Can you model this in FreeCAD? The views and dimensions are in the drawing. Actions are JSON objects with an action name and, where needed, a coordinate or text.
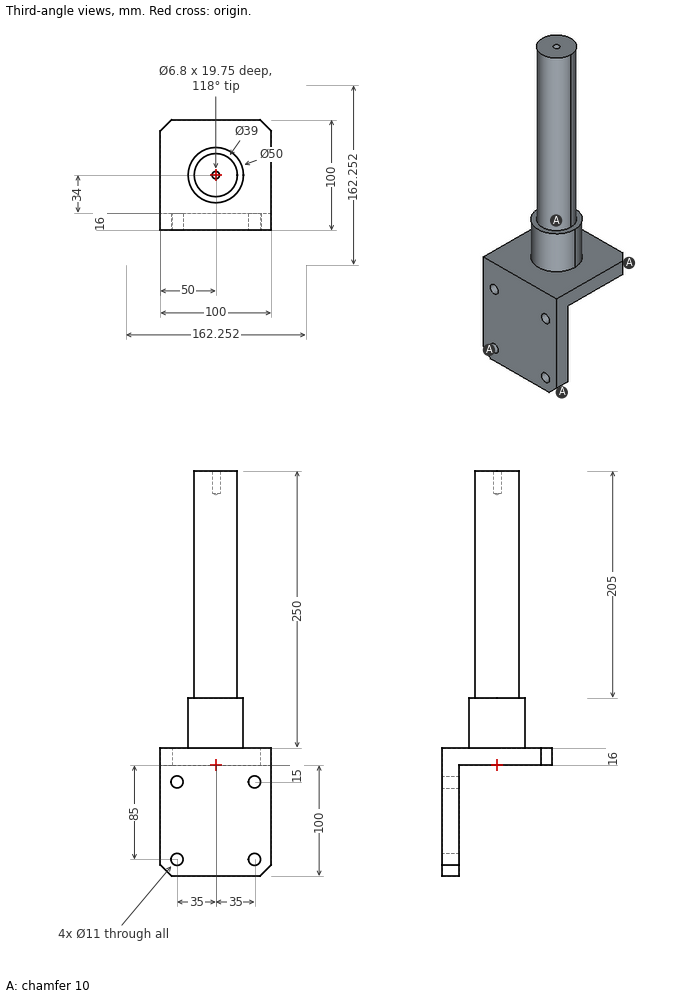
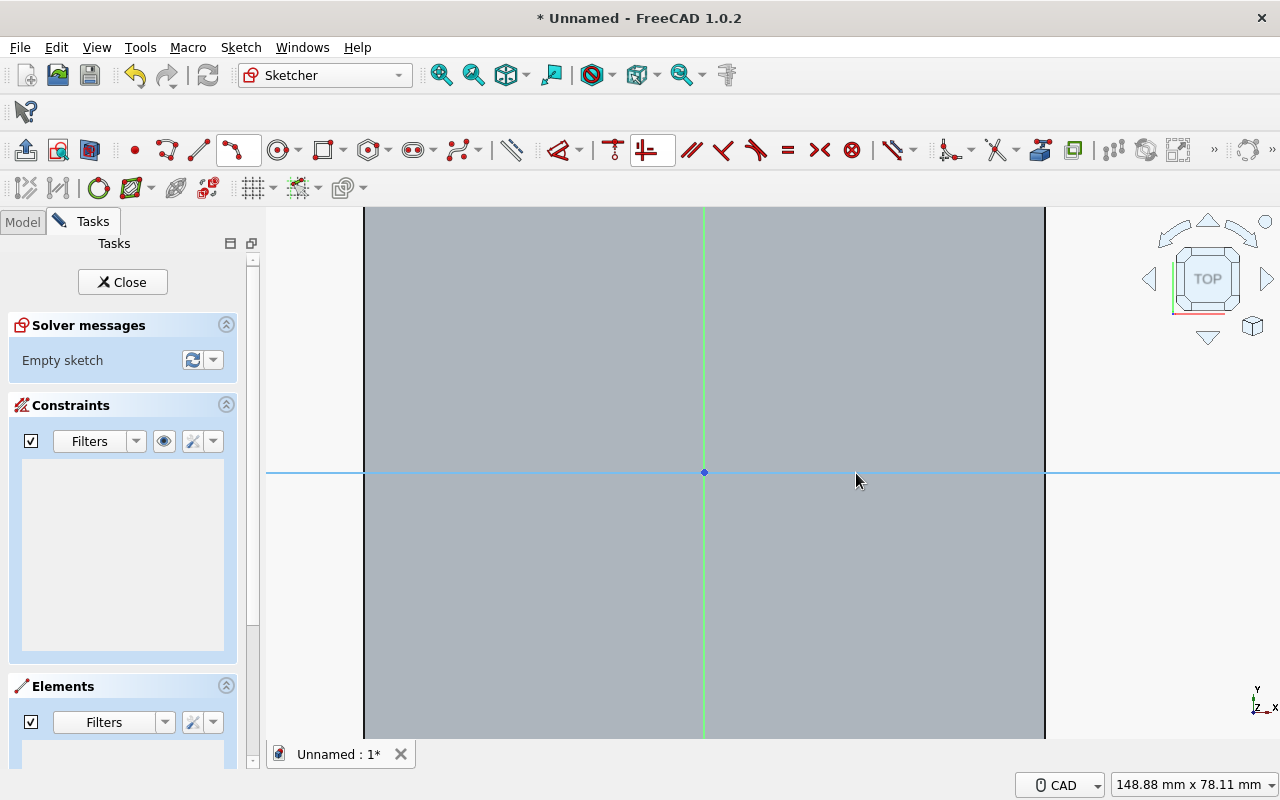
{"action": "left_click", "coordinate": [278, 150]}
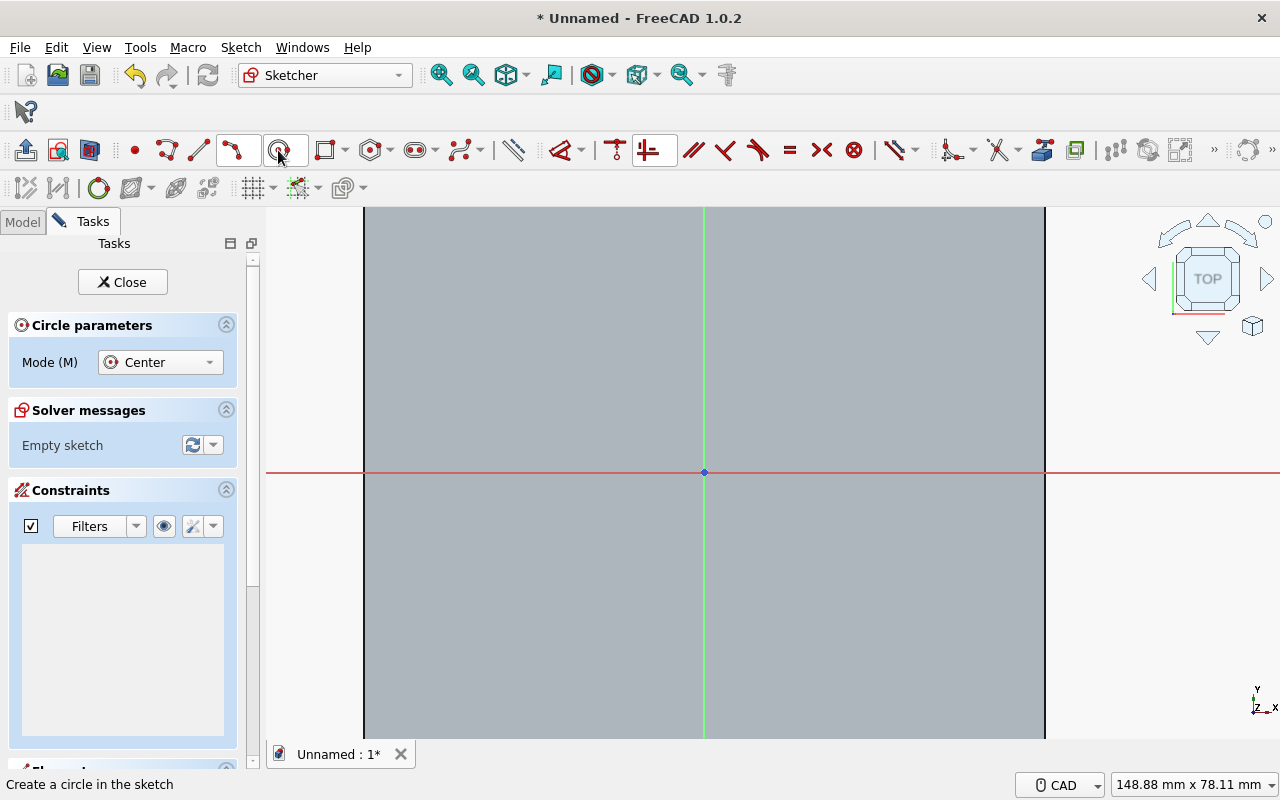
{"action": "left_click", "coordinate": [704, 473]}
{"action": "left_click", "coordinate": [825, 352]}
{"action": "key", "text": "Escape"}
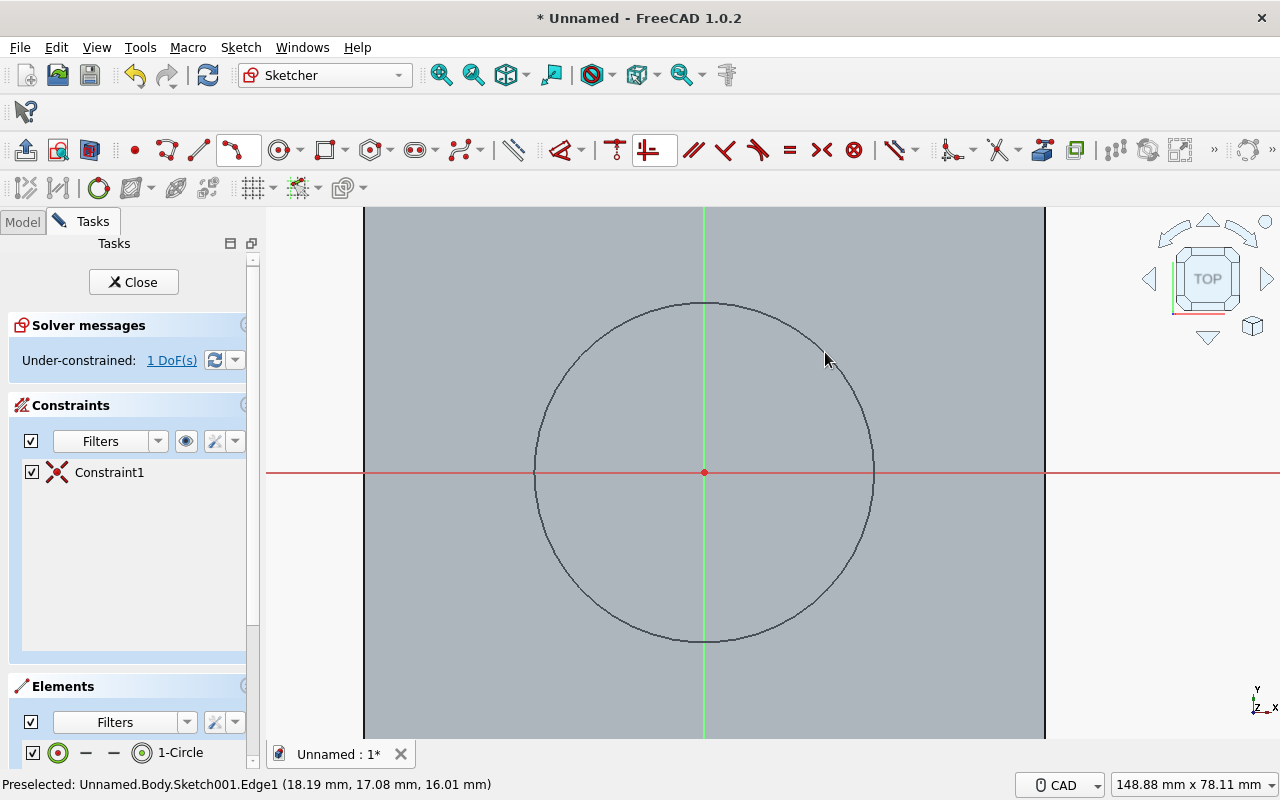
{"action": "left_click", "coordinate": [560, 150]}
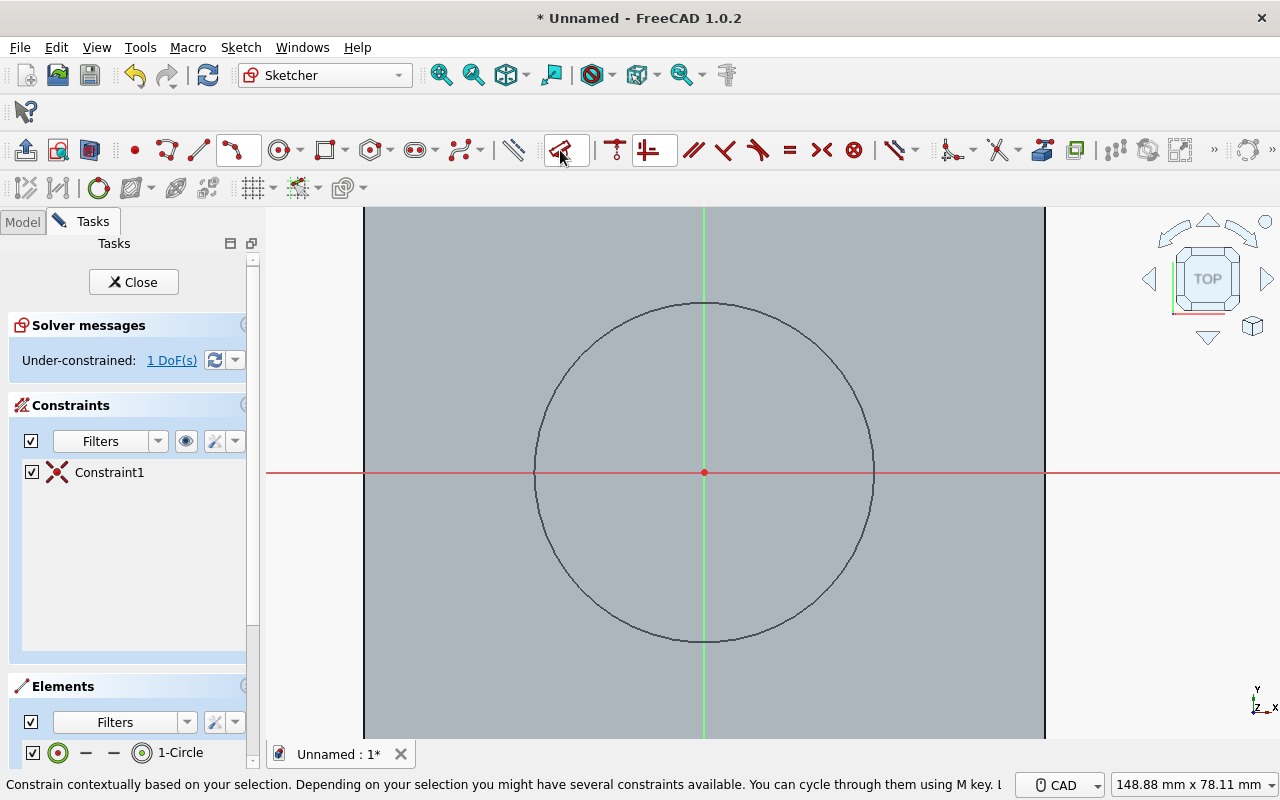
{"action": "left_click", "coordinate": [824, 352]}
{"action": "left_click", "coordinate": [847, 329]}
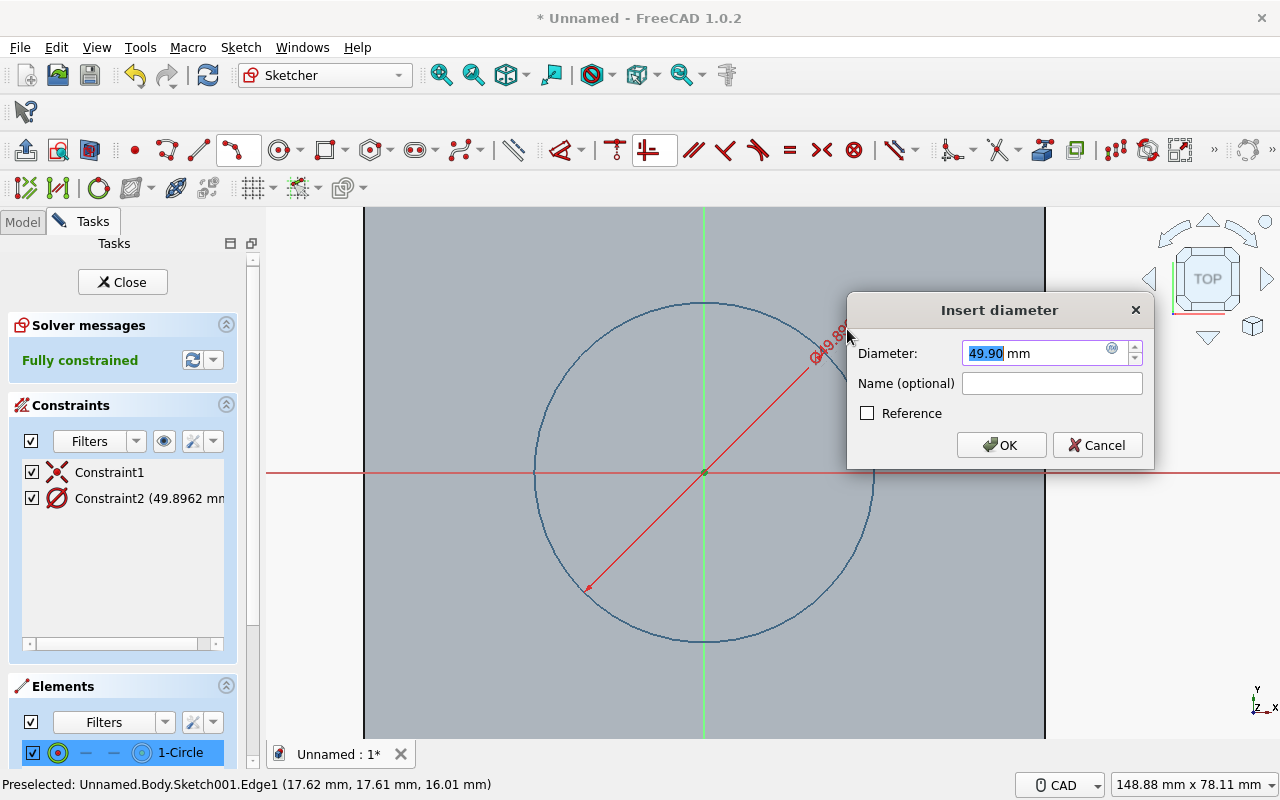
{"action": "type", "text": "50"}
{"action": "key", "text": "Return"}
{"action": "key", "text": "Escape"}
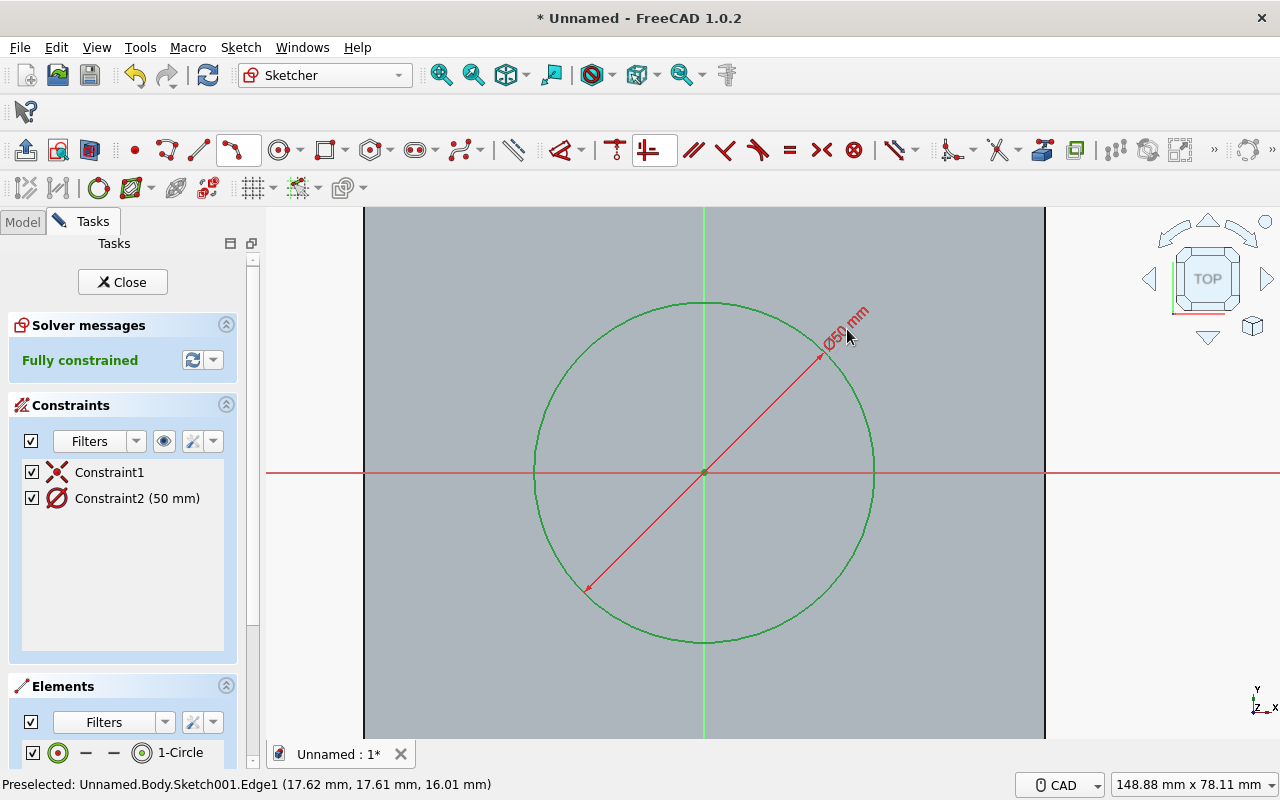
{"action": "left_click", "coordinate": [123, 282]}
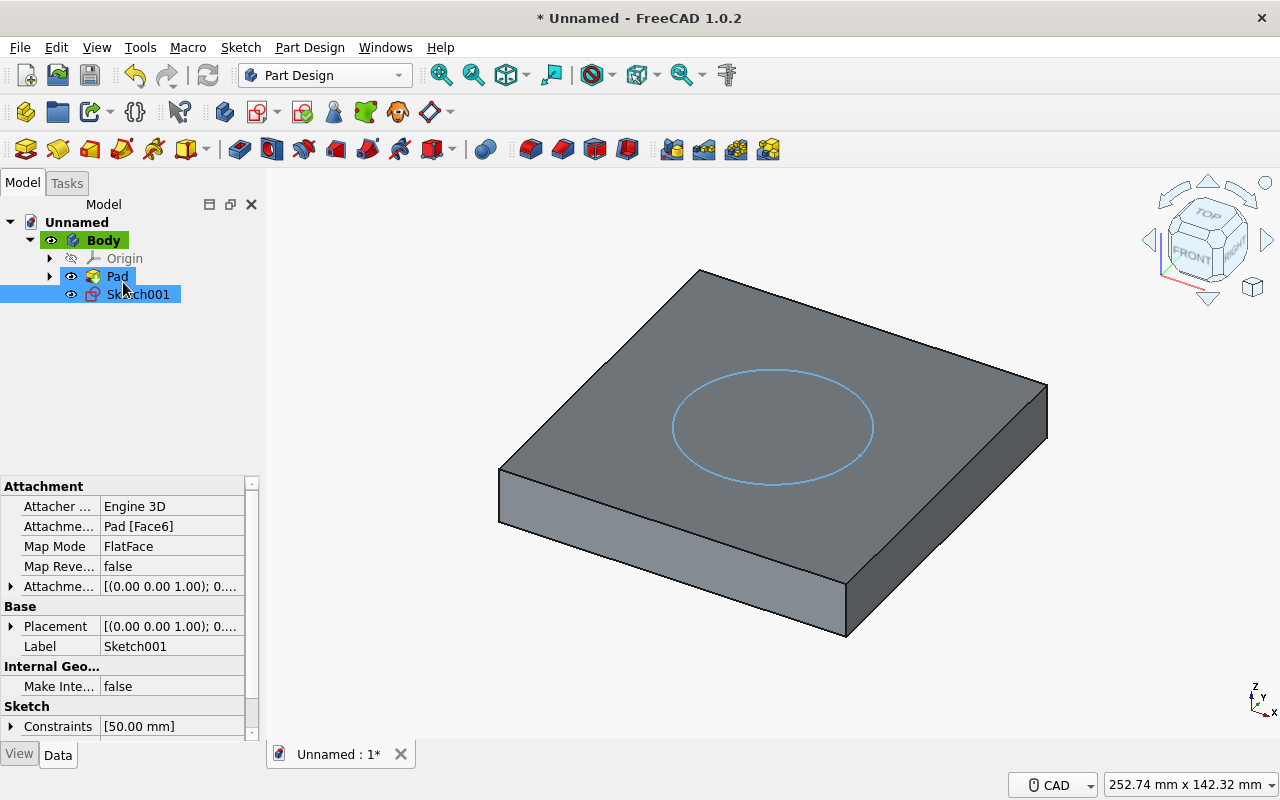
{"action": "left_click", "coordinate": [26, 150]}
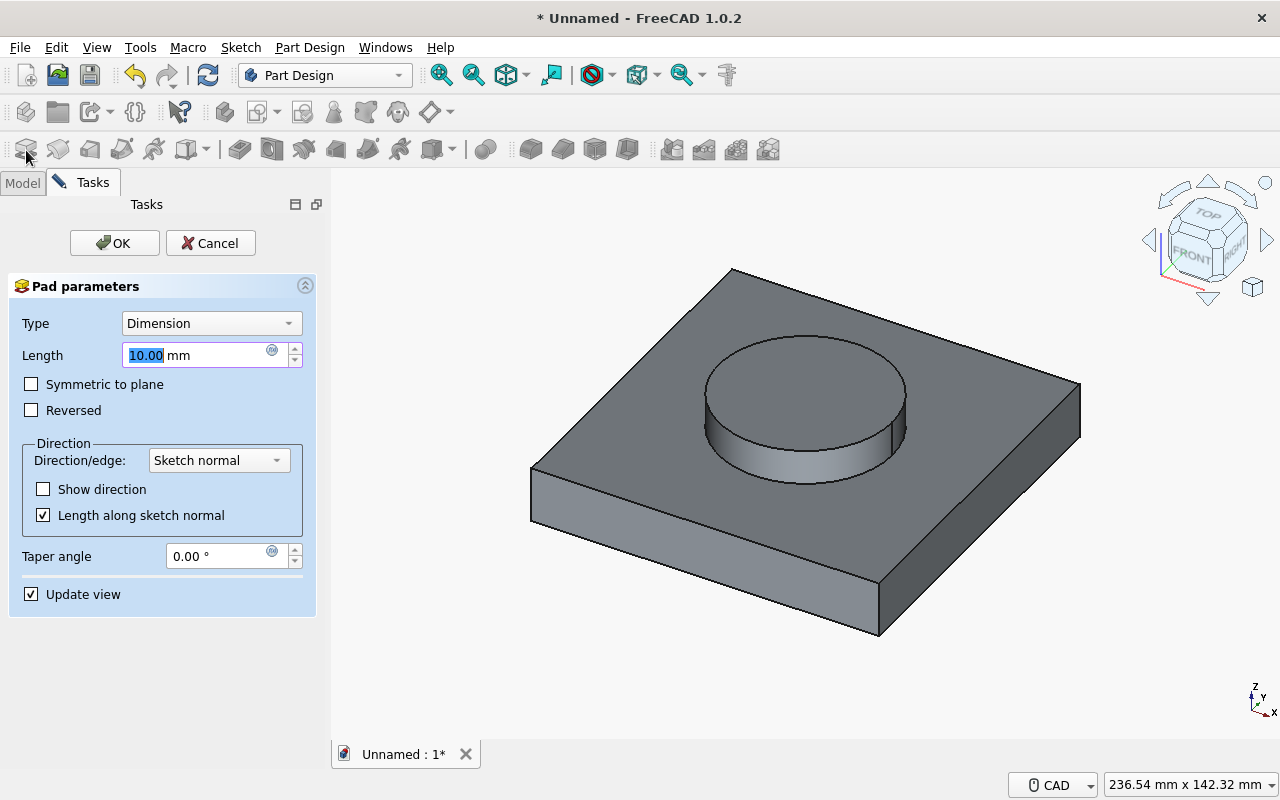
{"action": "type", "text": "250"}
{"action": "key", "text": "Tab"}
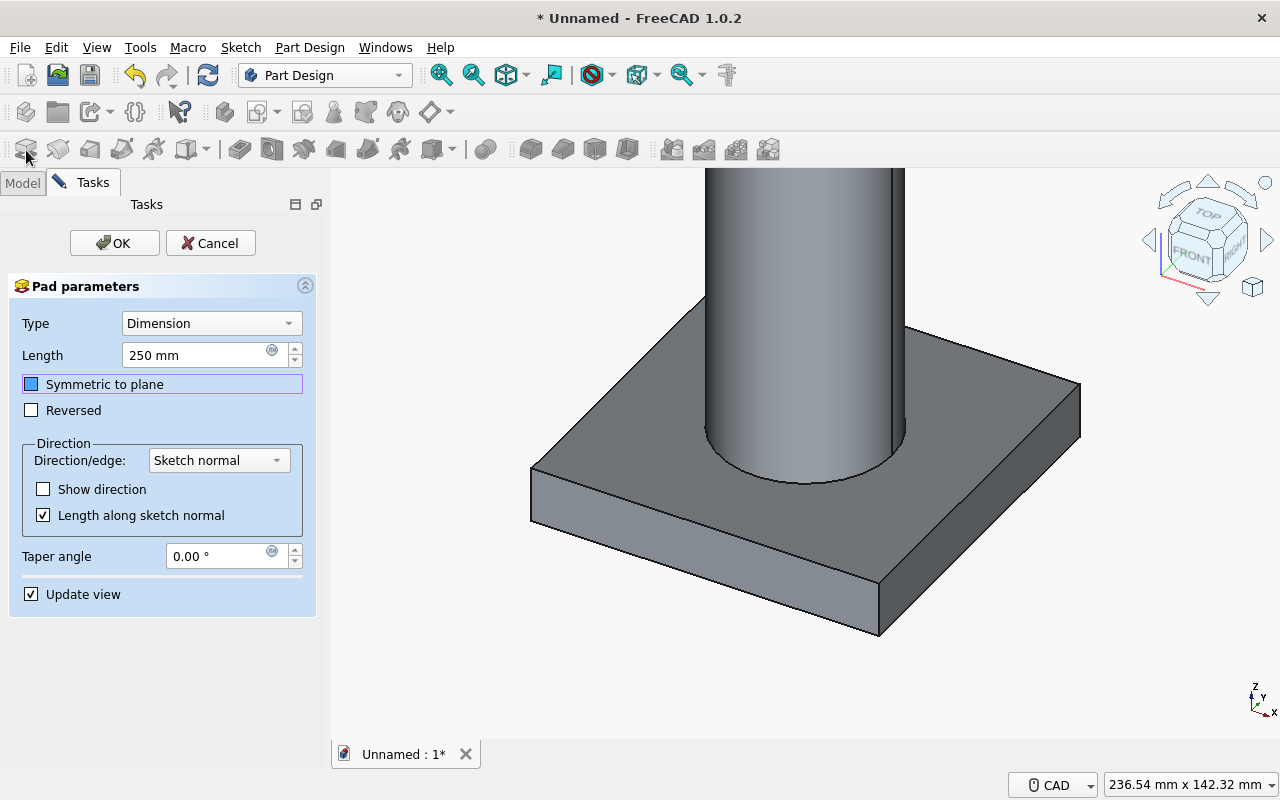
{"action": "left_click", "coordinate": [115, 243]}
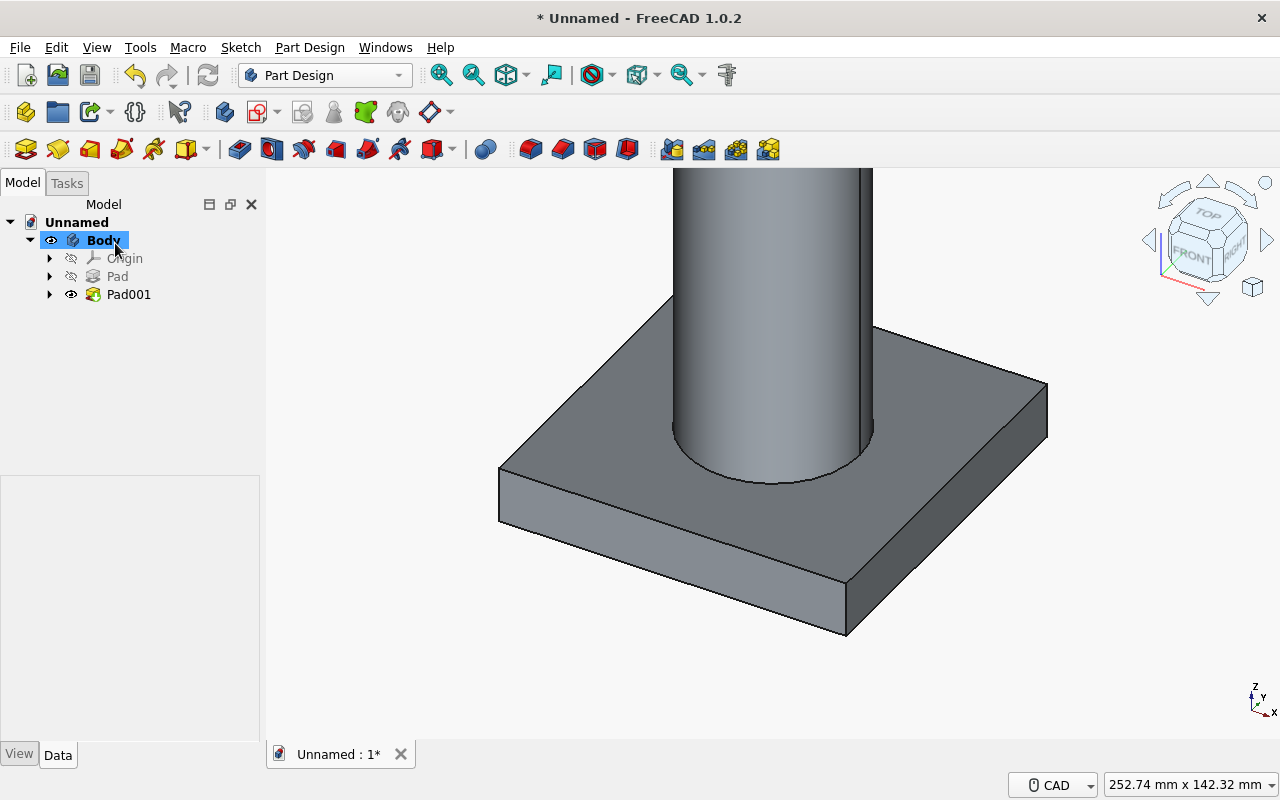
{"action": "left_click", "coordinate": [442, 76]}